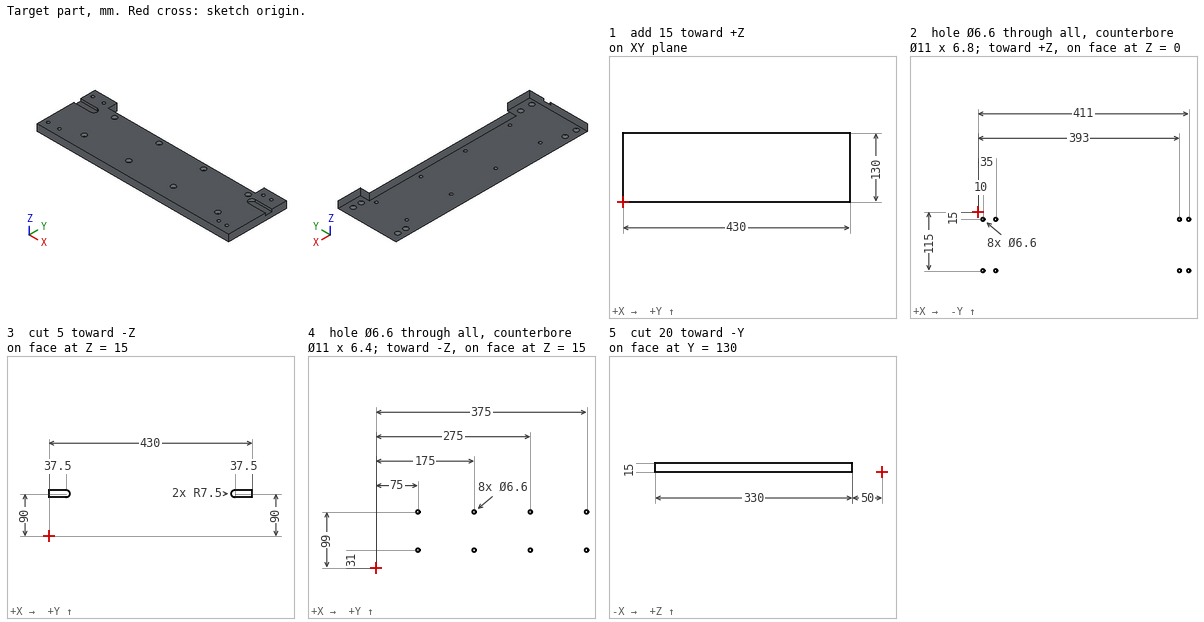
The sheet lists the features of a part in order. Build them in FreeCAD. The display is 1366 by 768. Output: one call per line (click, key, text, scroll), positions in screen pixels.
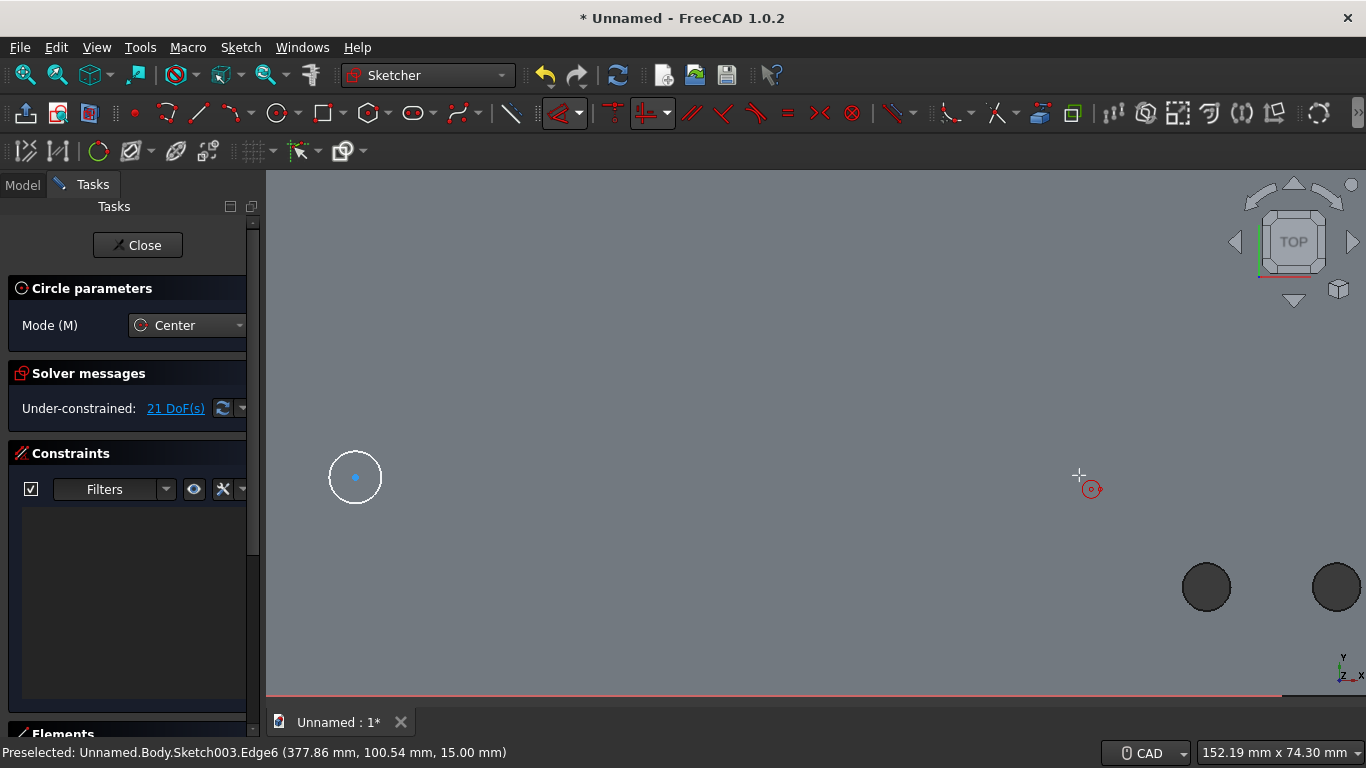
scroll(1079, 475, down, 7)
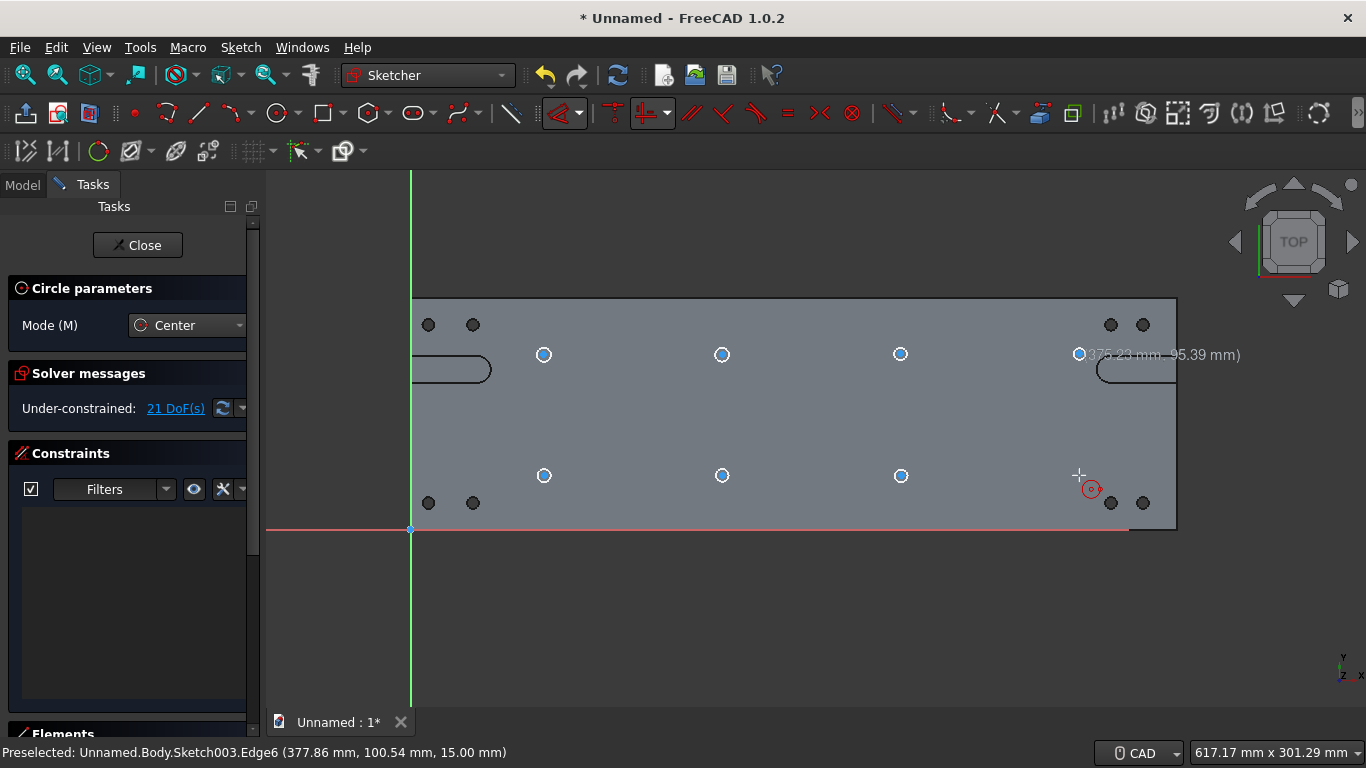
click(1079, 475)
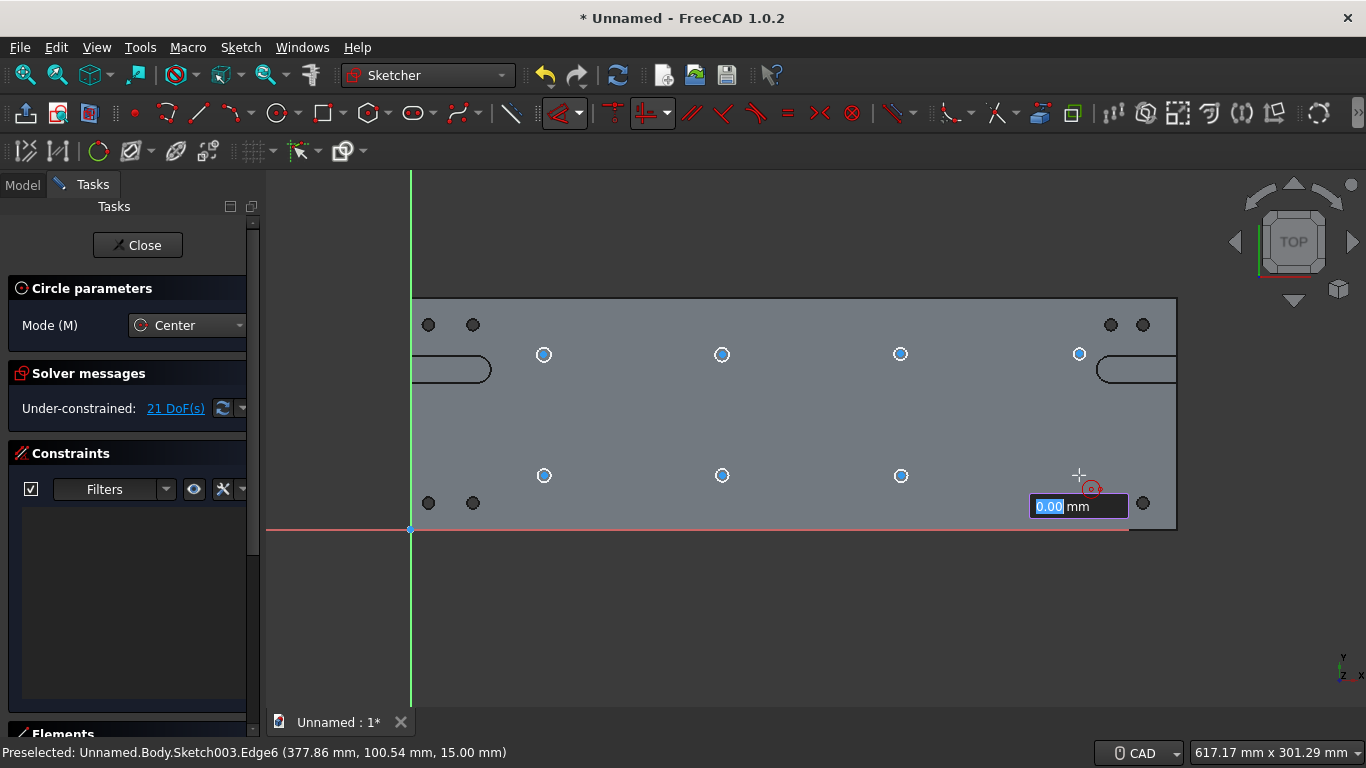
scroll(1083, 470, up, 5)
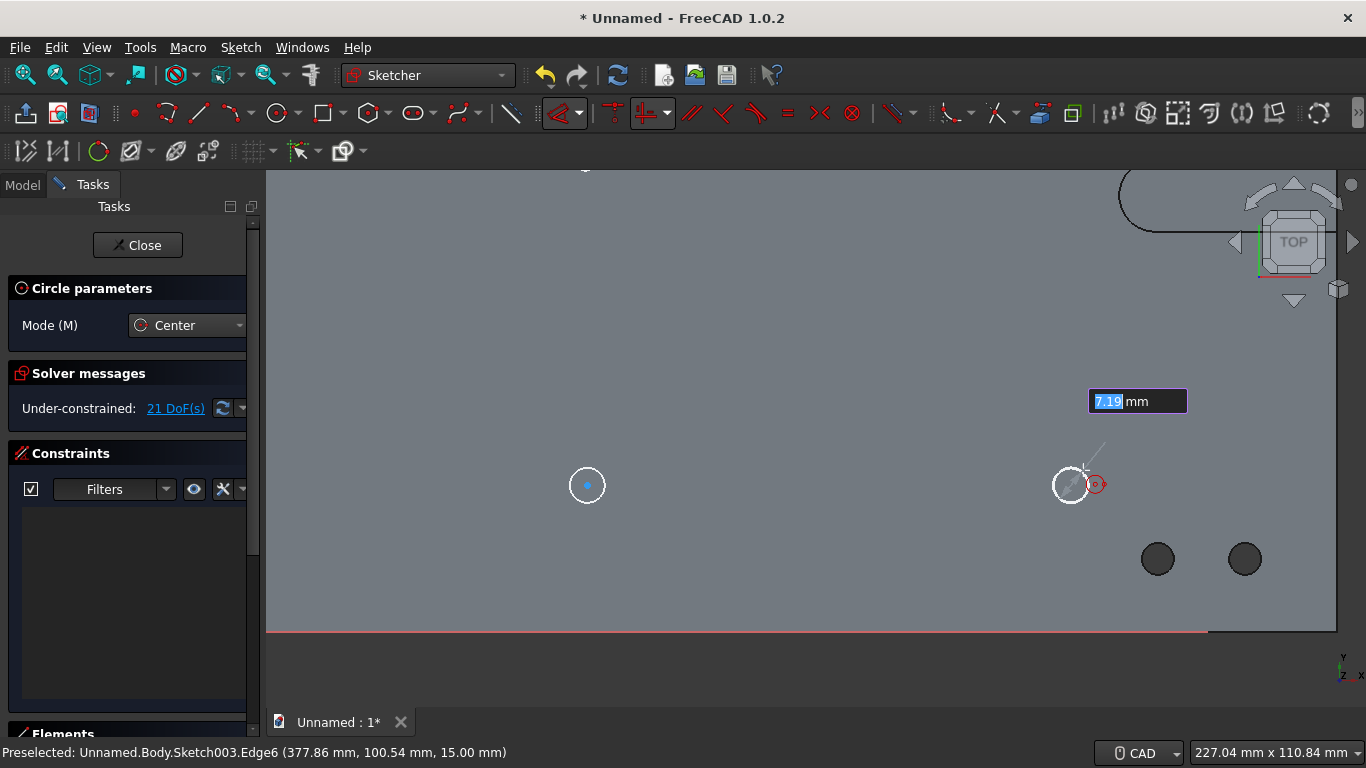
click(1082, 470)
key(Escape)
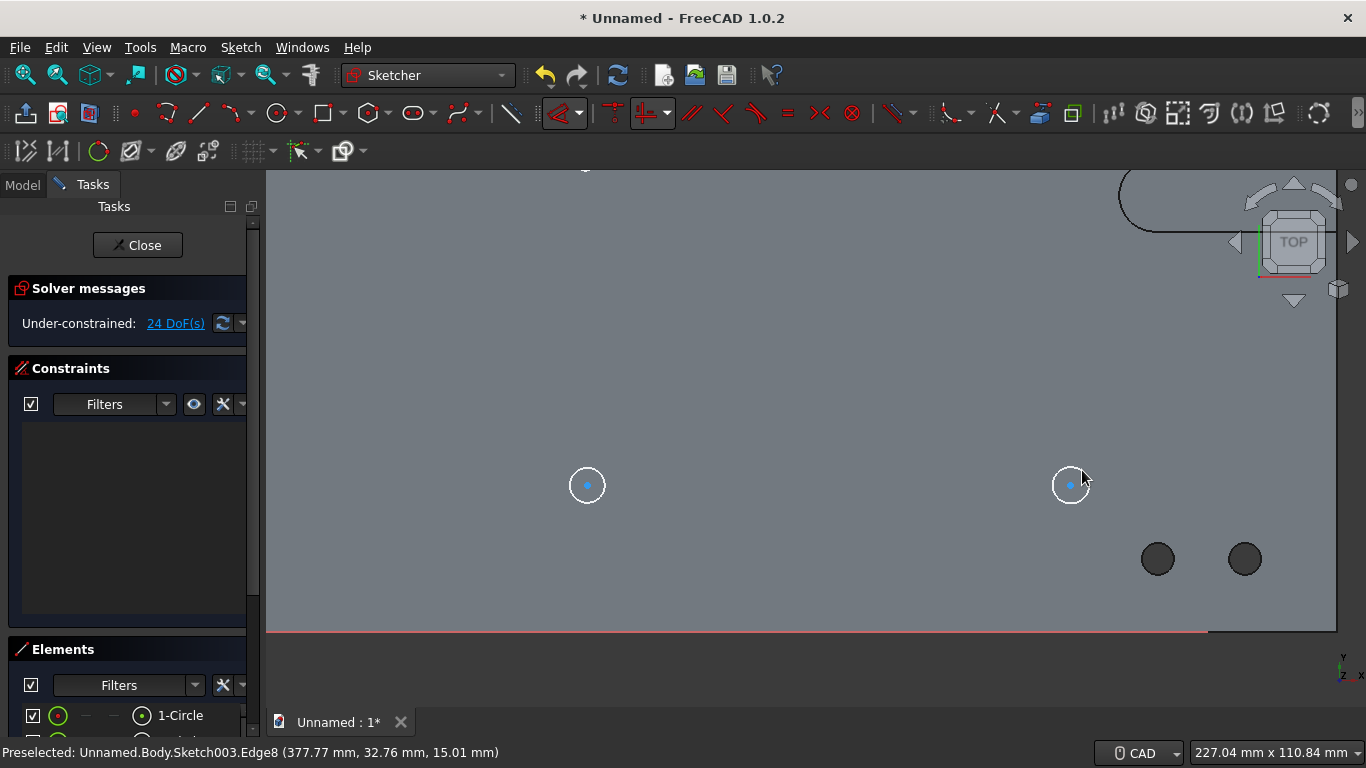
scroll(1083, 470, down, 5)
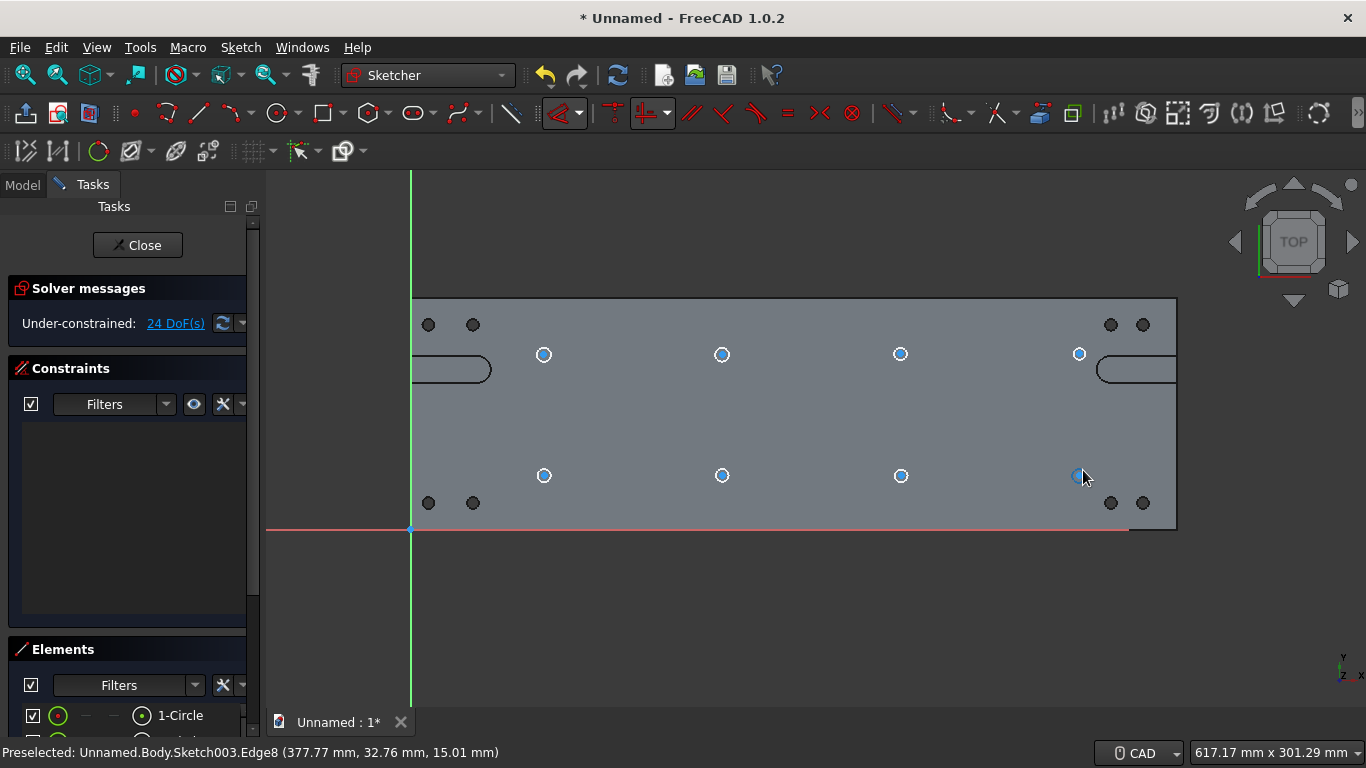
scroll(549, 350, up, 4)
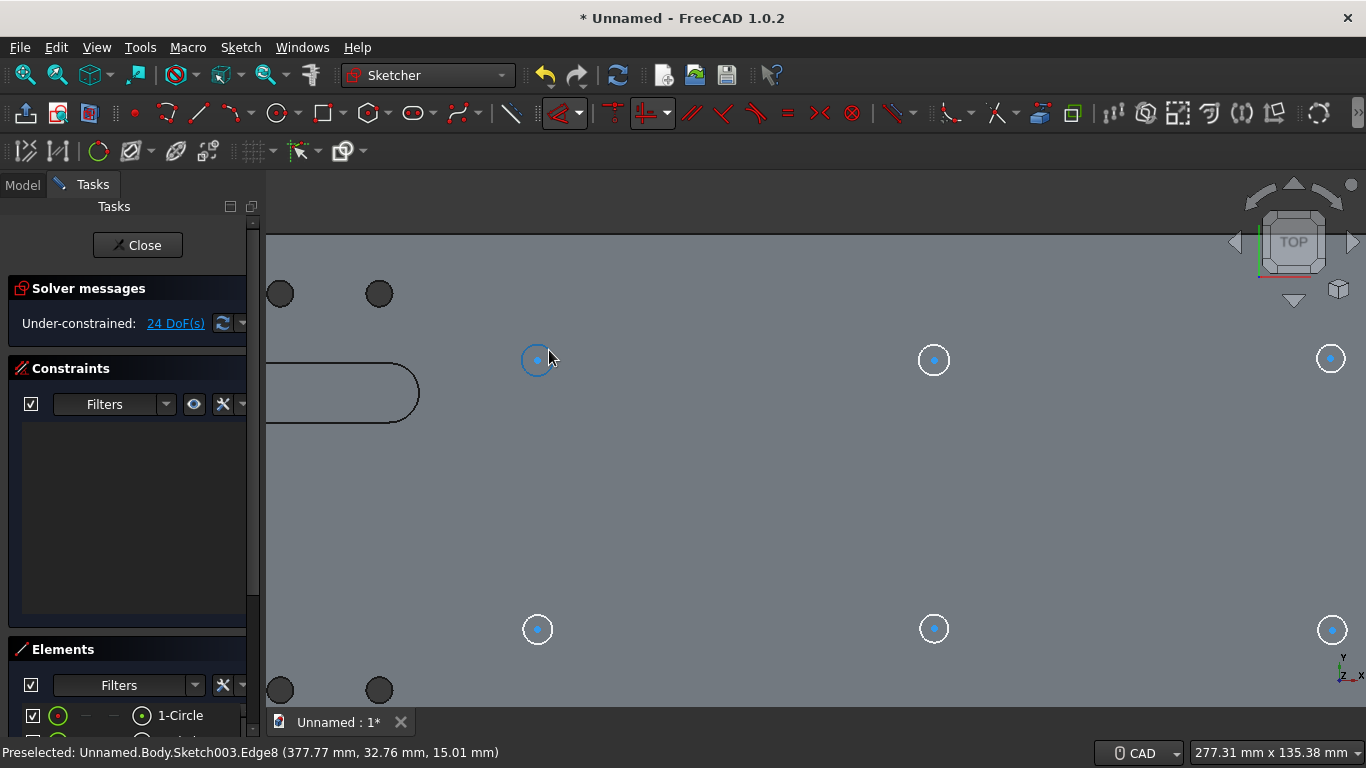
click(548, 349)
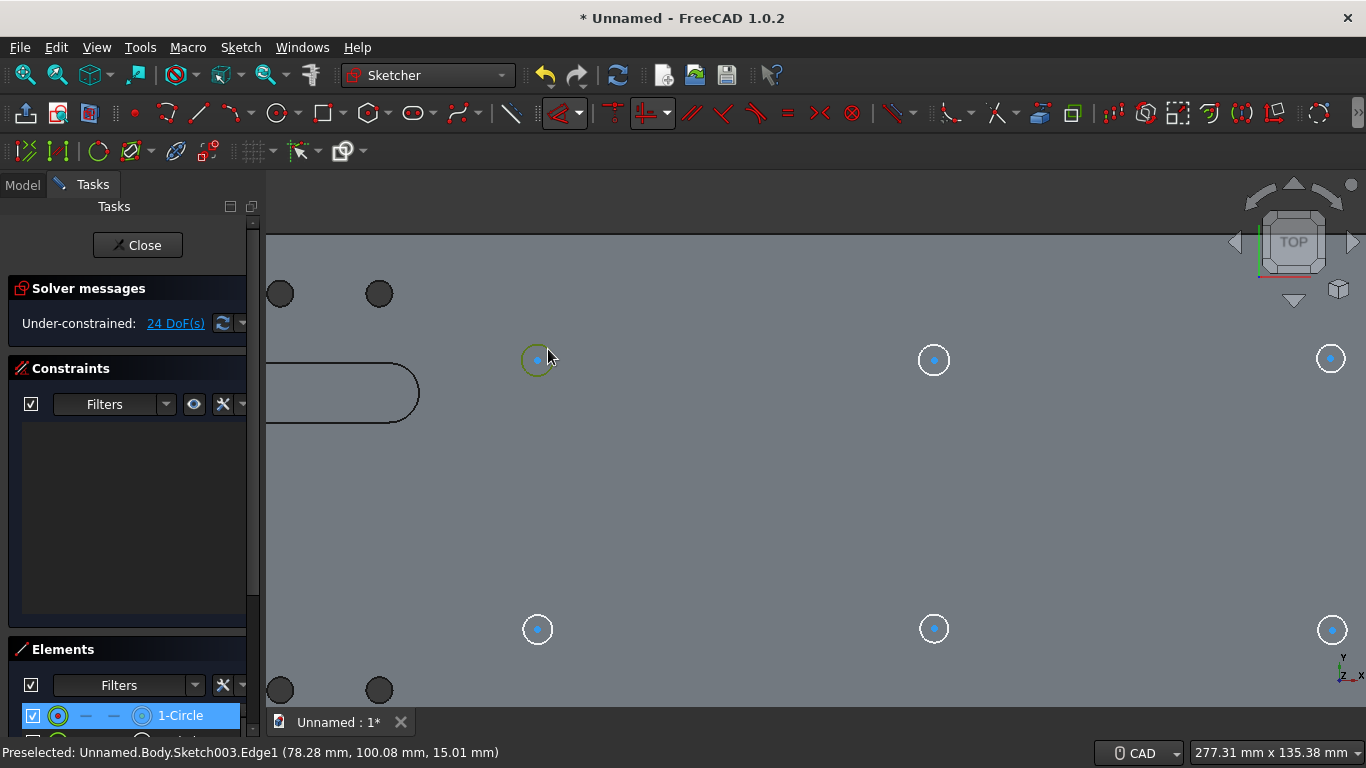
click(945, 349)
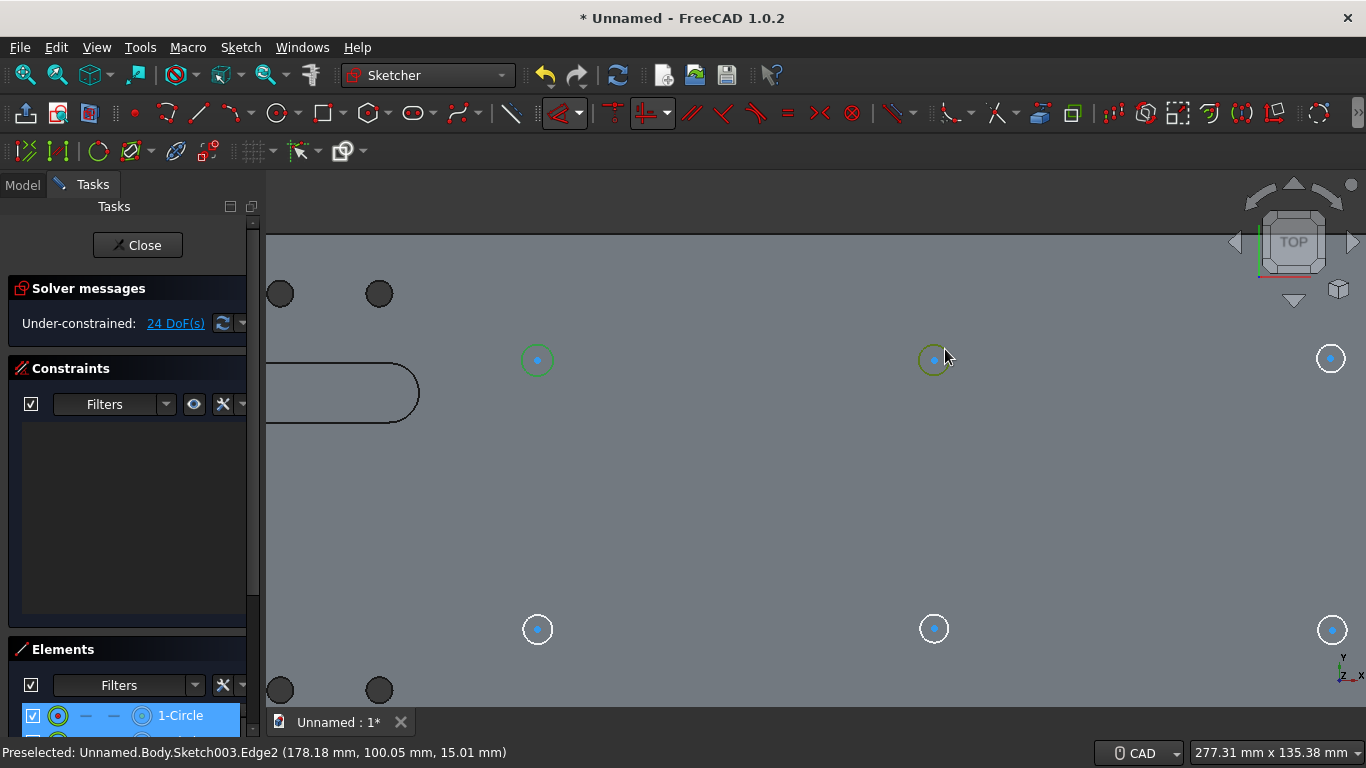
click(548, 619)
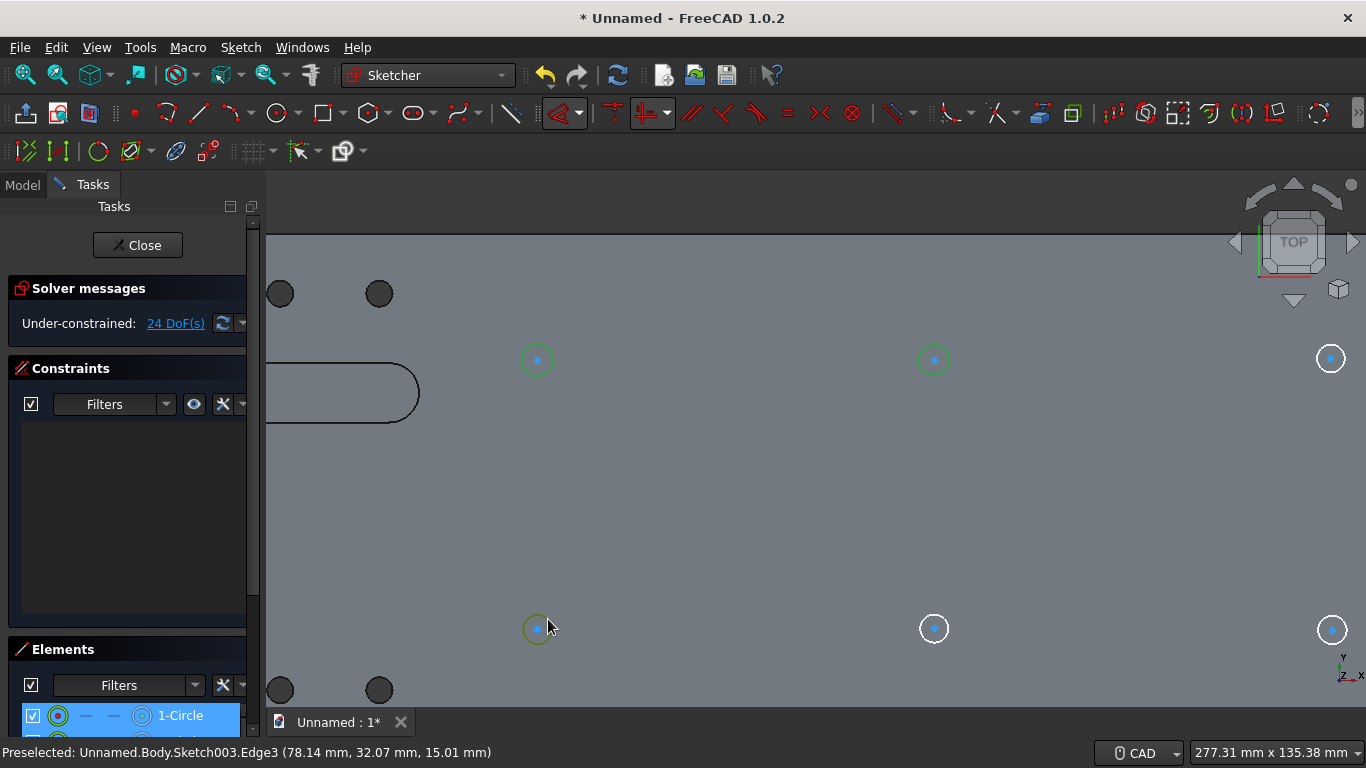
click(944, 619)